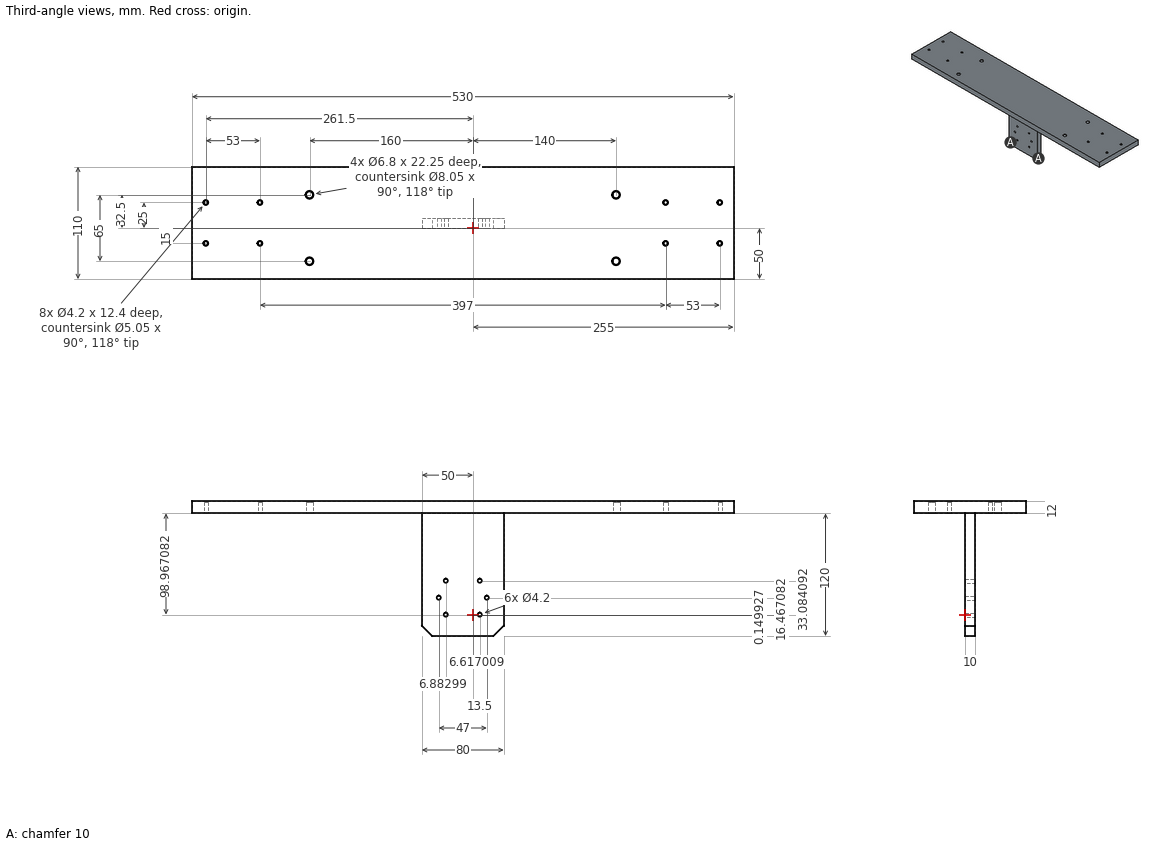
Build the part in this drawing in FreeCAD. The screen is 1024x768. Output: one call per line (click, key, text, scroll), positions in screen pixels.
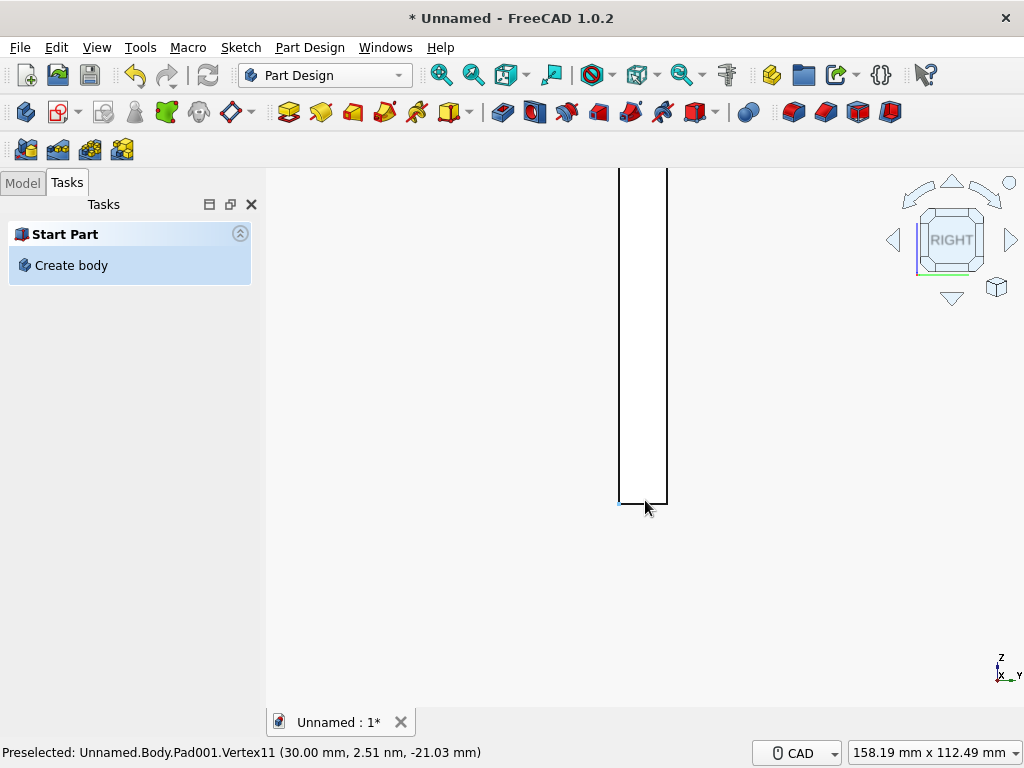
click(643, 503)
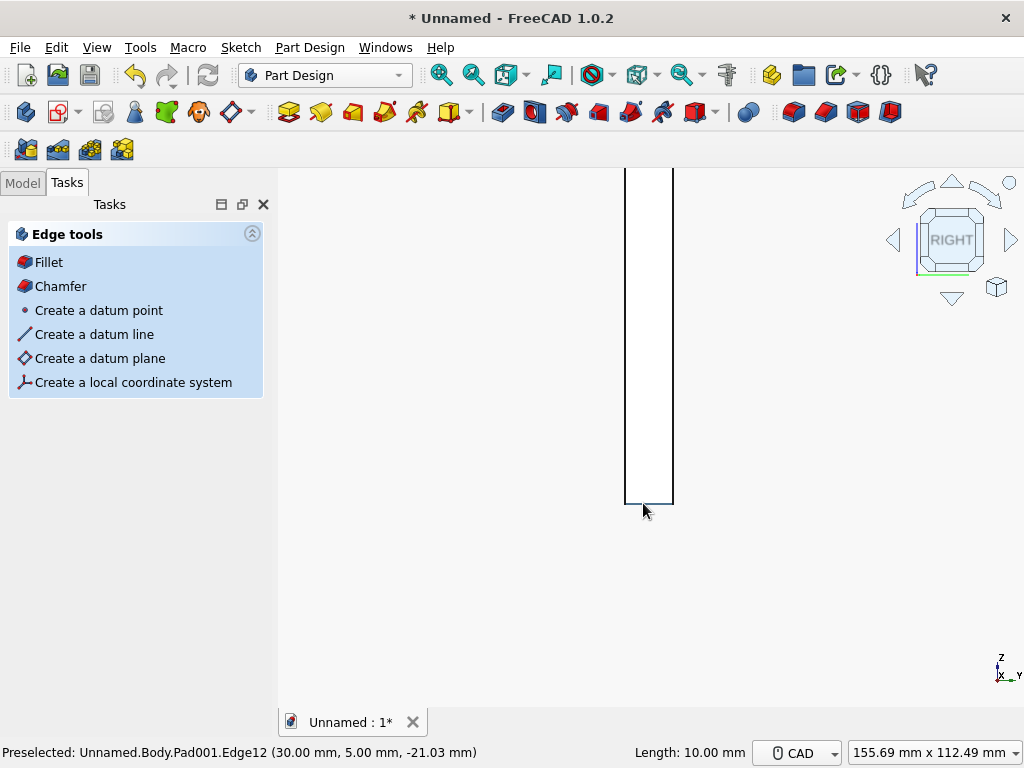
key(v)
key(f)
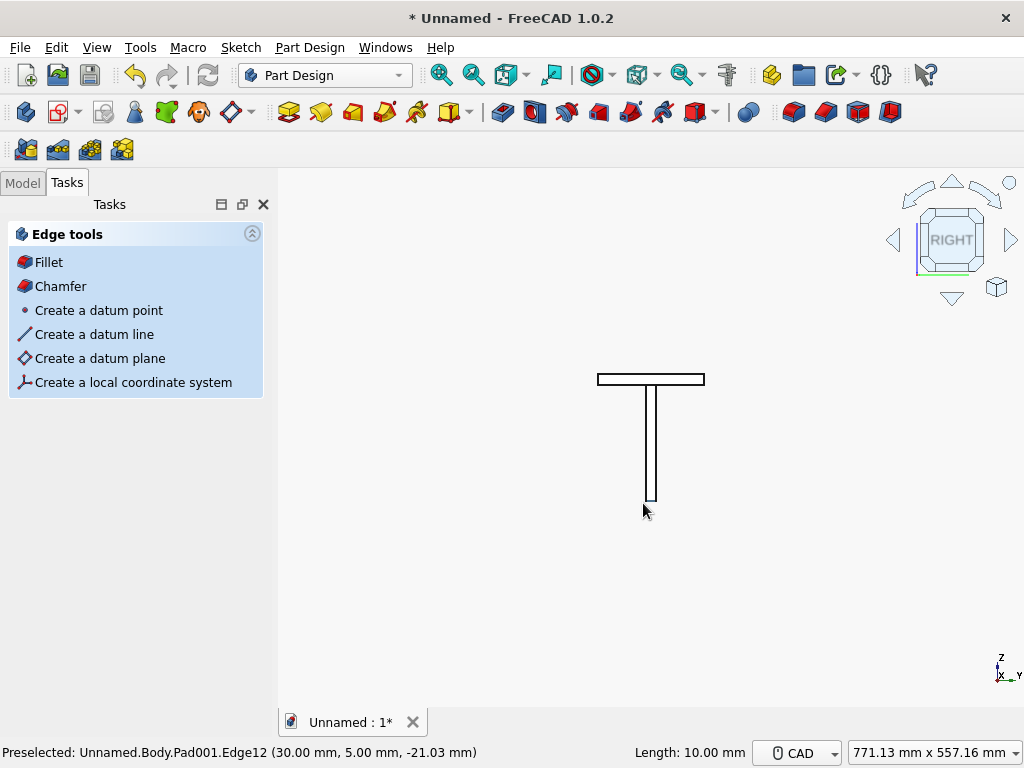
key(5)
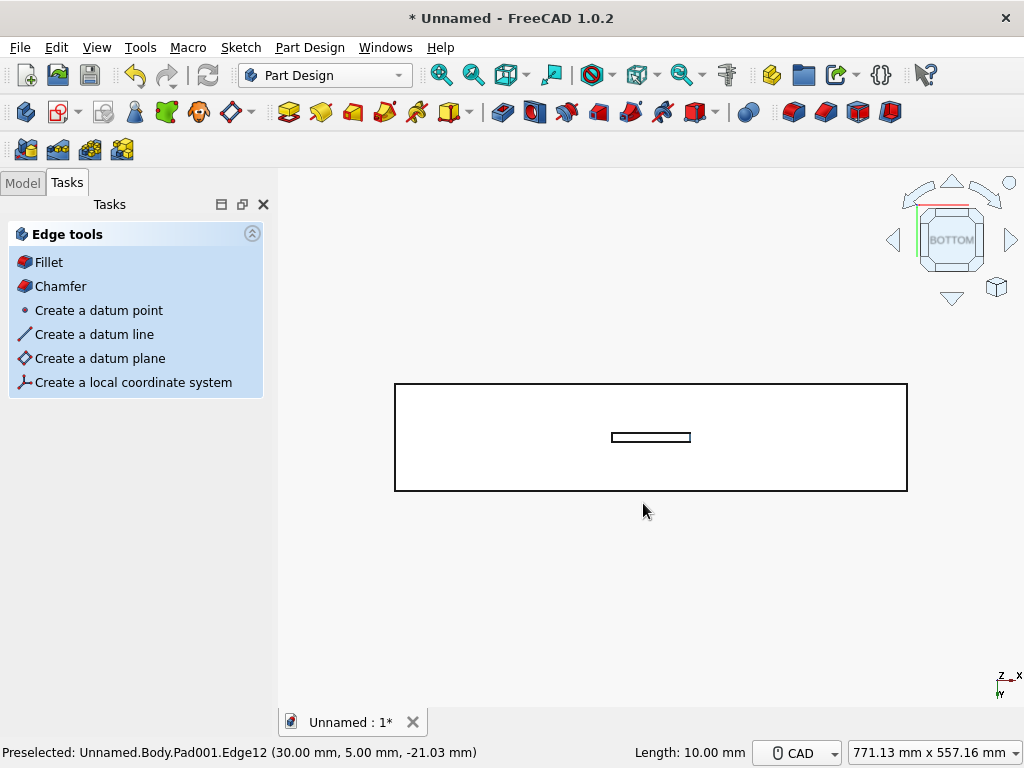
click(612, 438, ctrl)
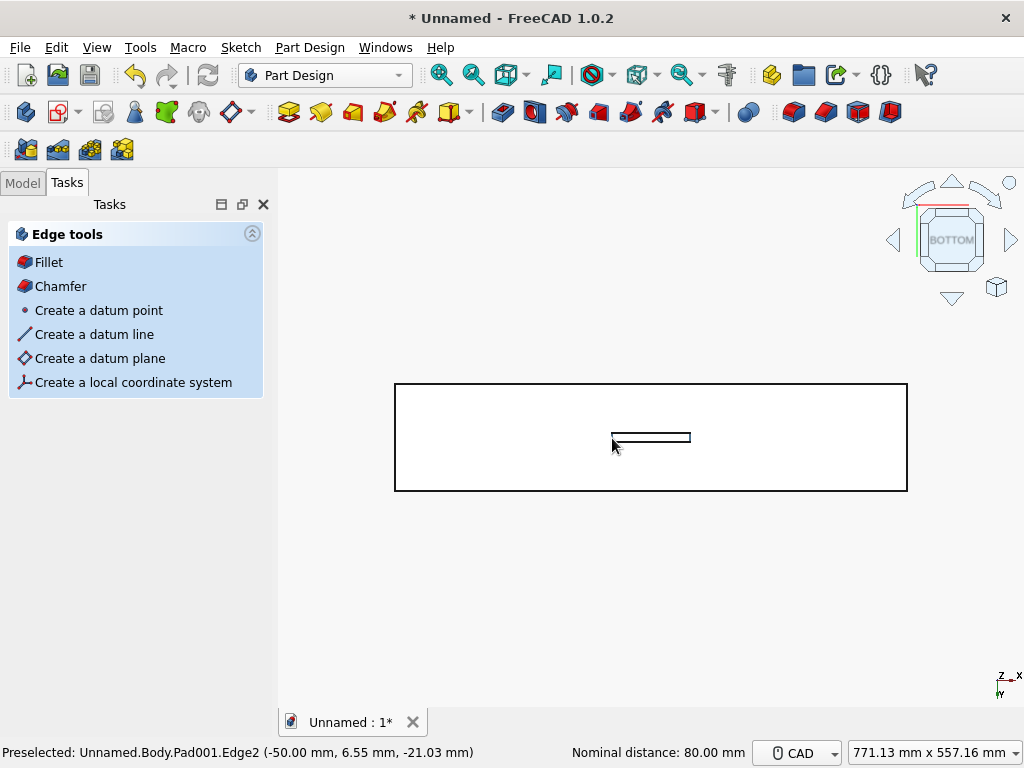
click(826, 112)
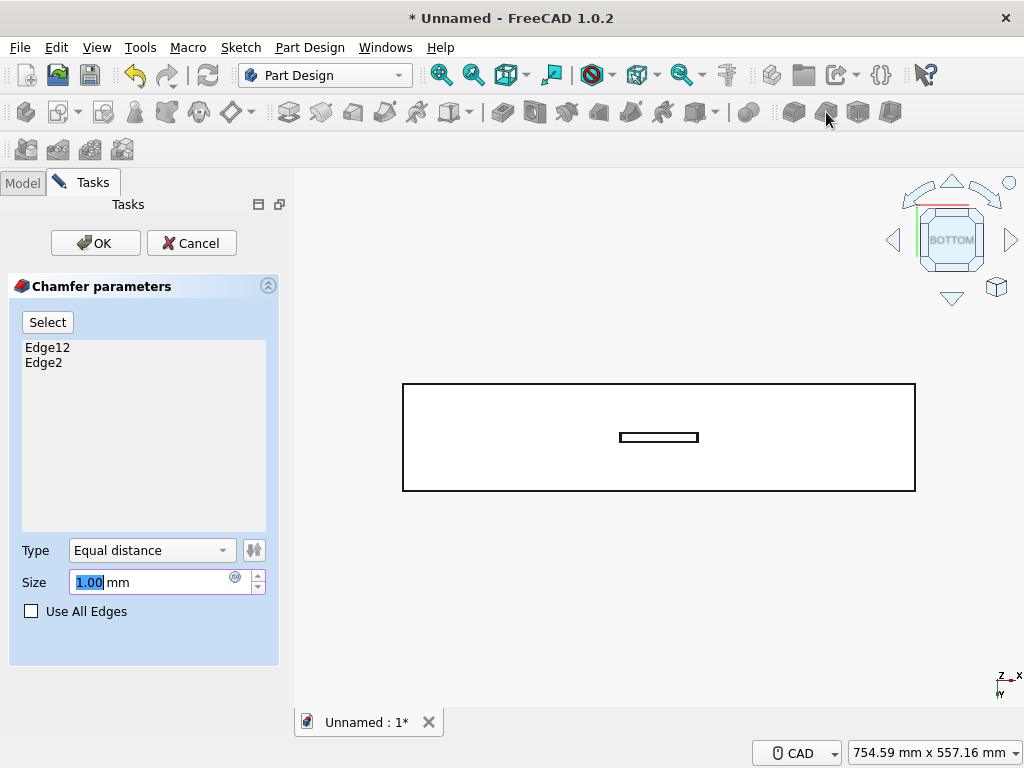
text(10)
key(Tab)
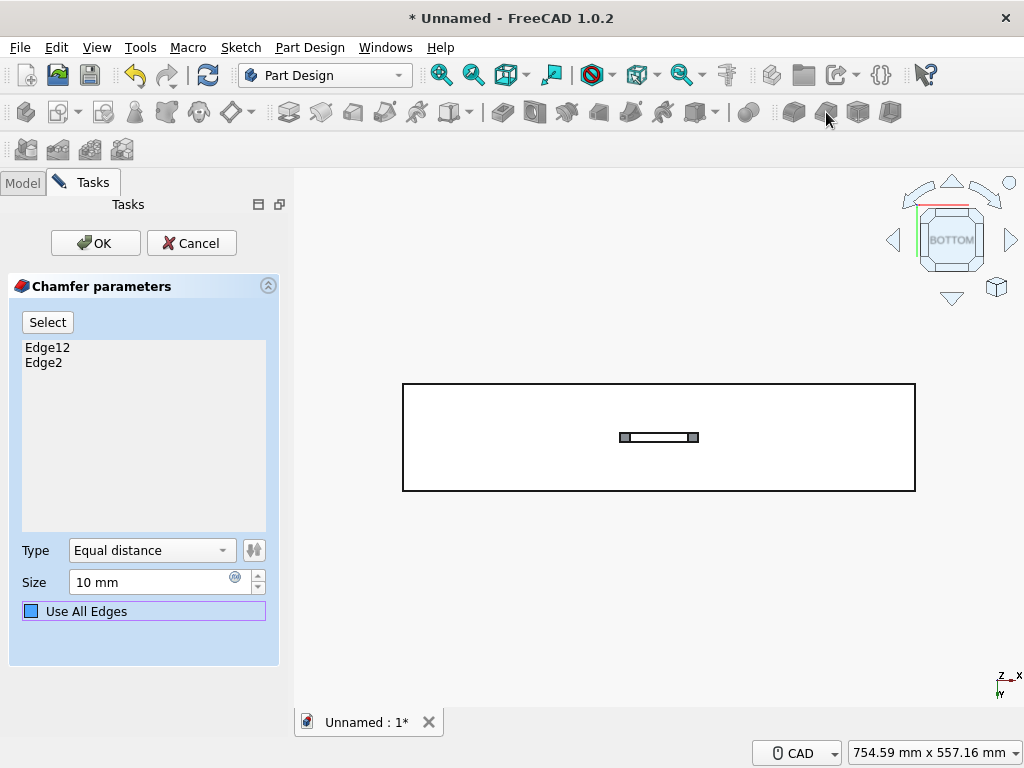
click(96, 243)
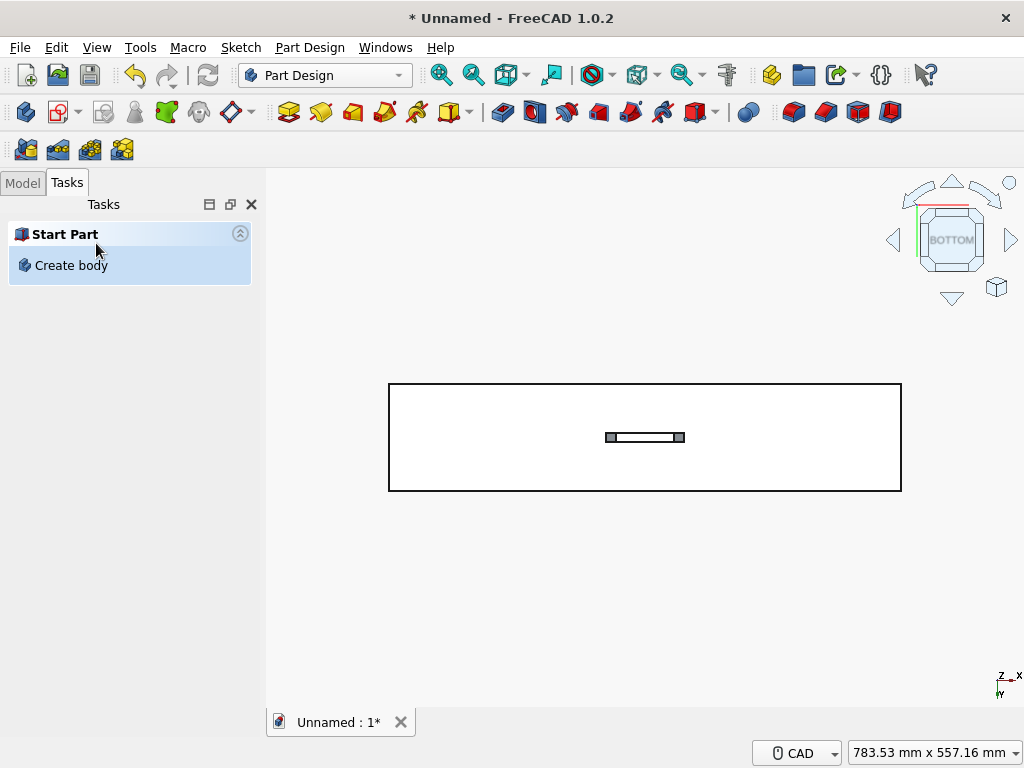
key(4)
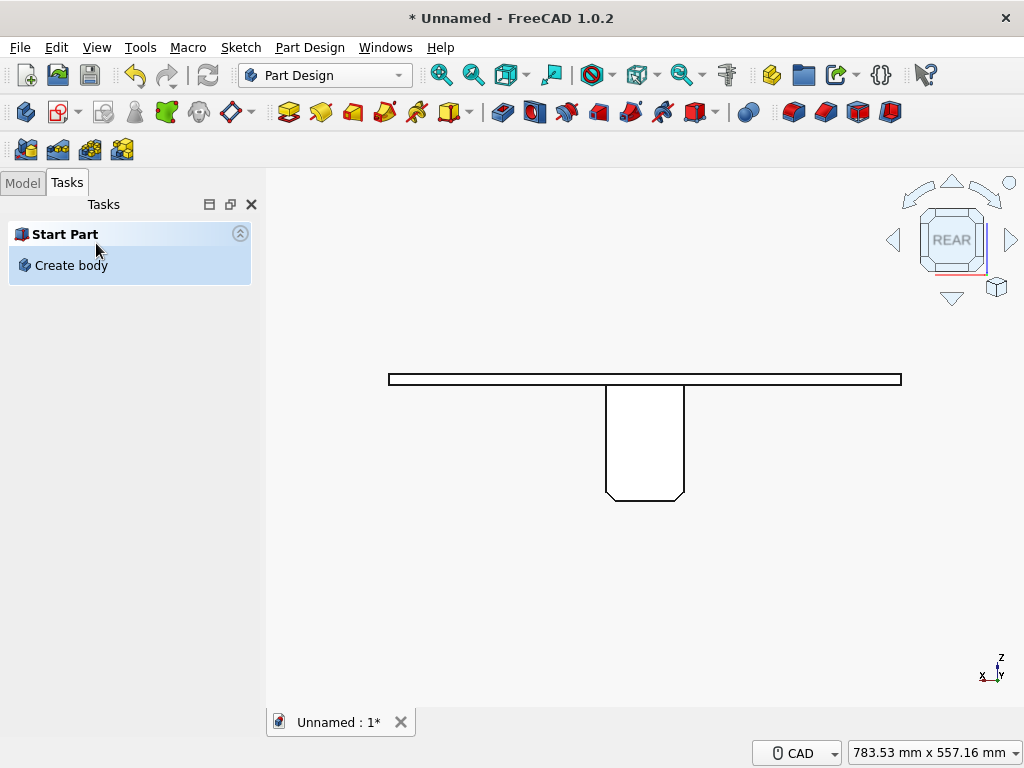
click(645, 426)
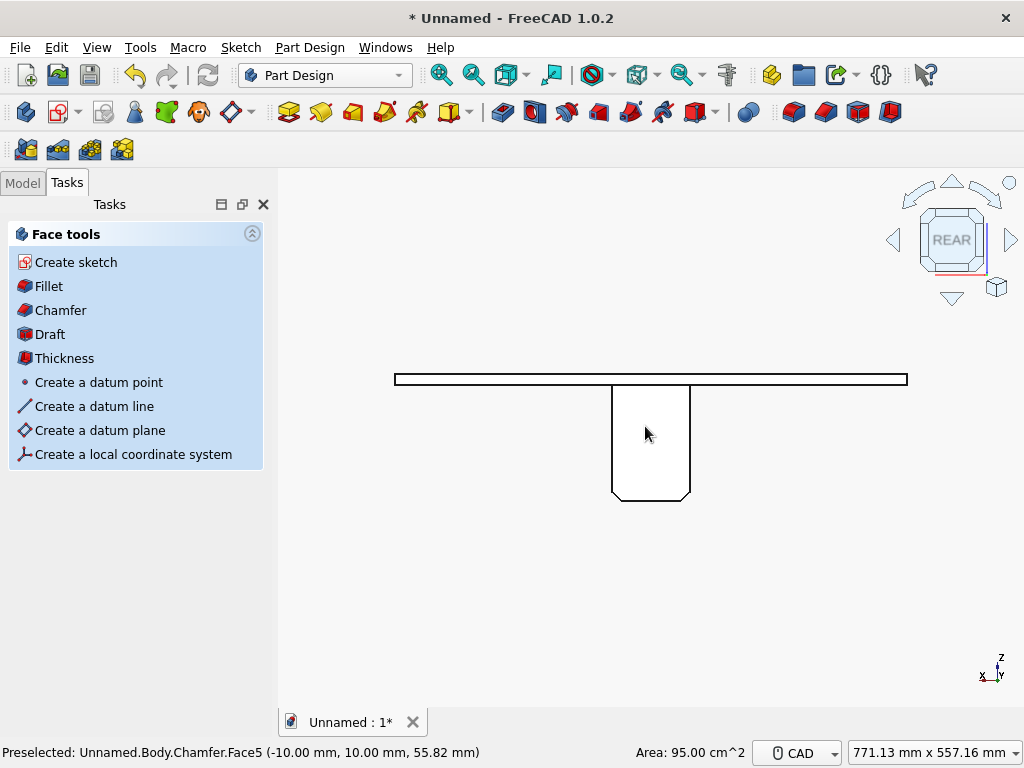
click(58, 112)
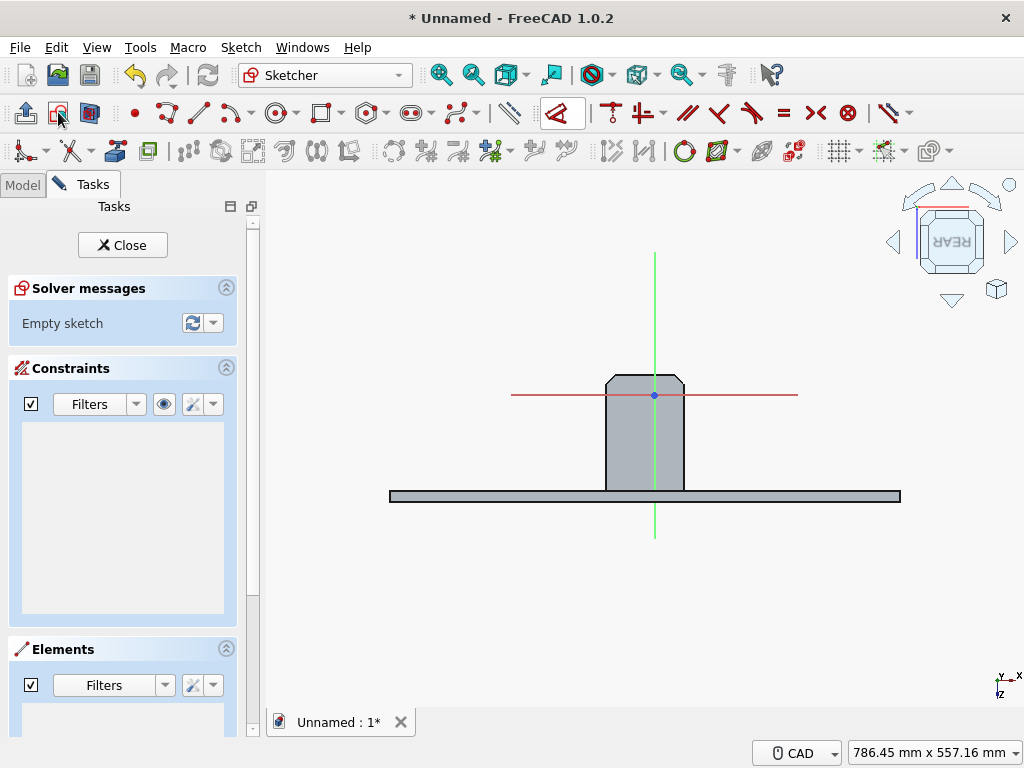
click(90, 114)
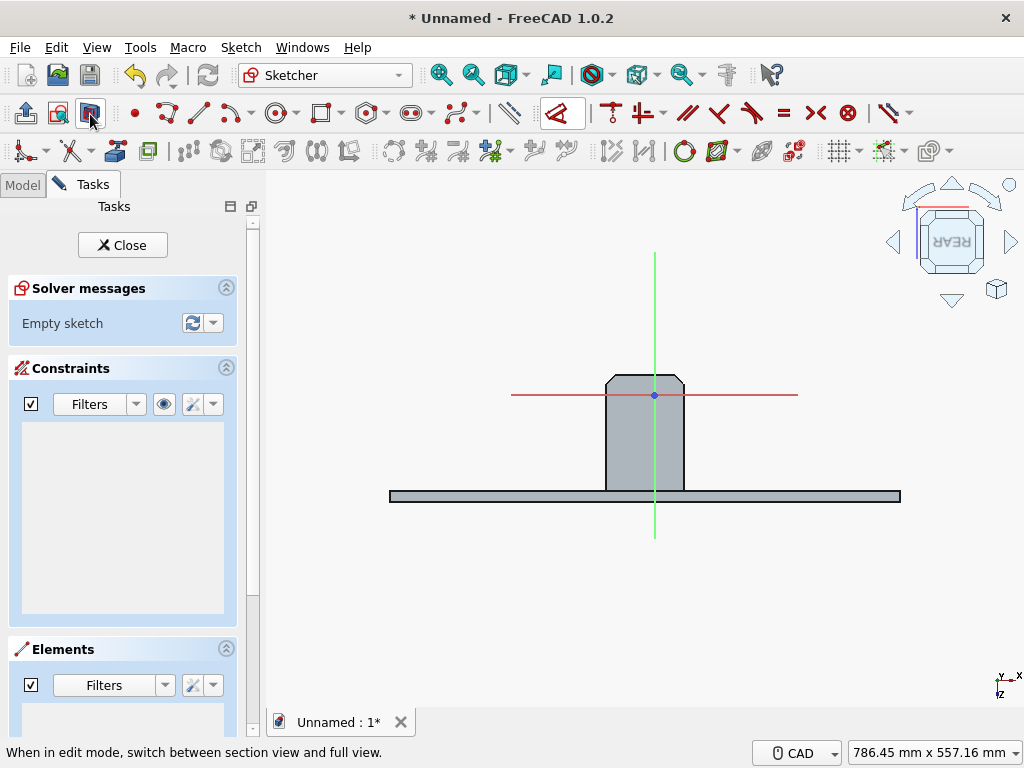
scroll(656, 407, up, 10)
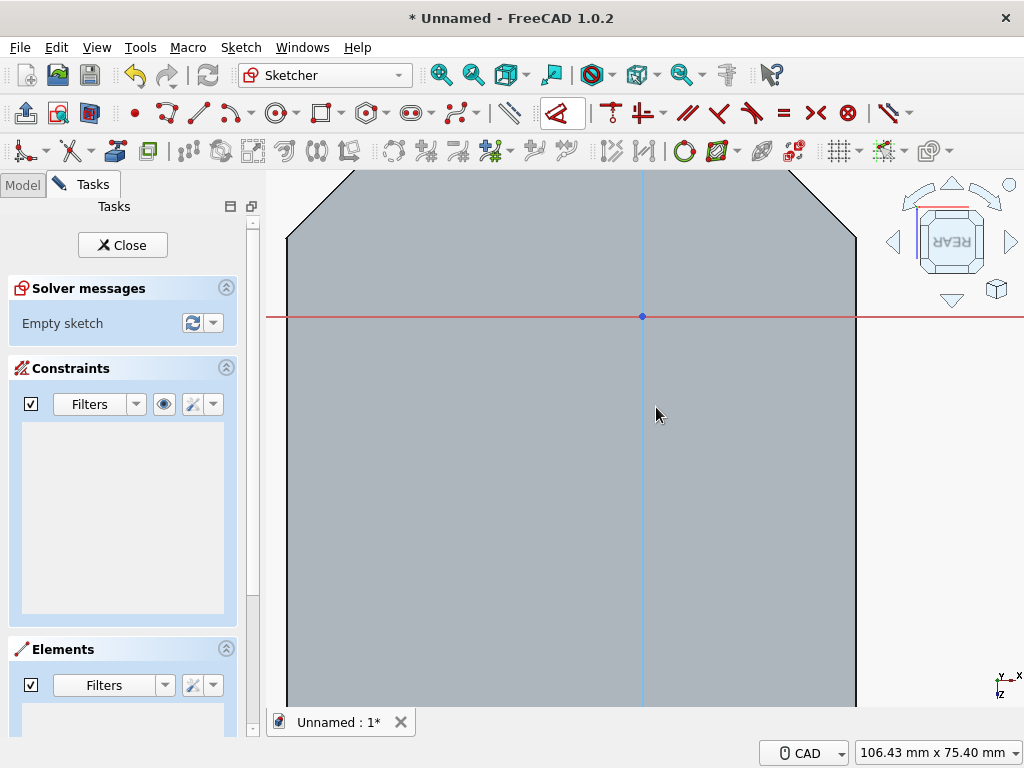
key(g)
key(c)